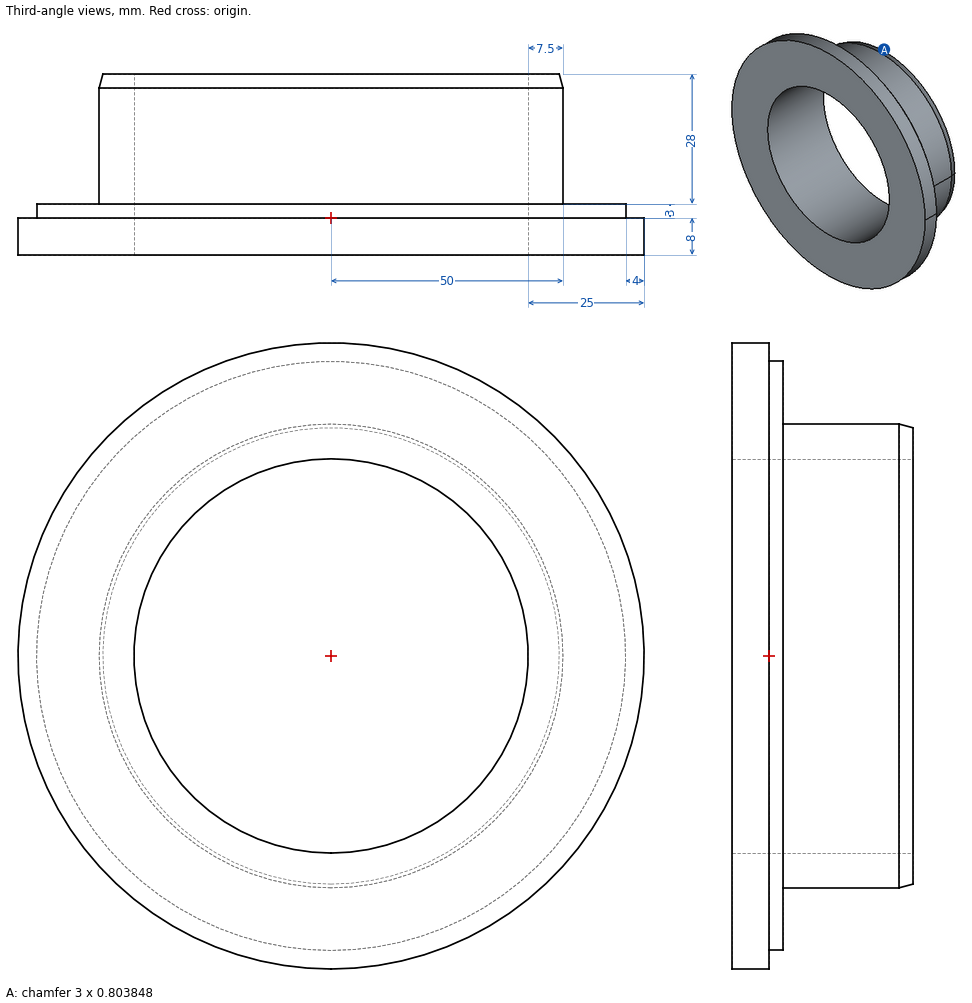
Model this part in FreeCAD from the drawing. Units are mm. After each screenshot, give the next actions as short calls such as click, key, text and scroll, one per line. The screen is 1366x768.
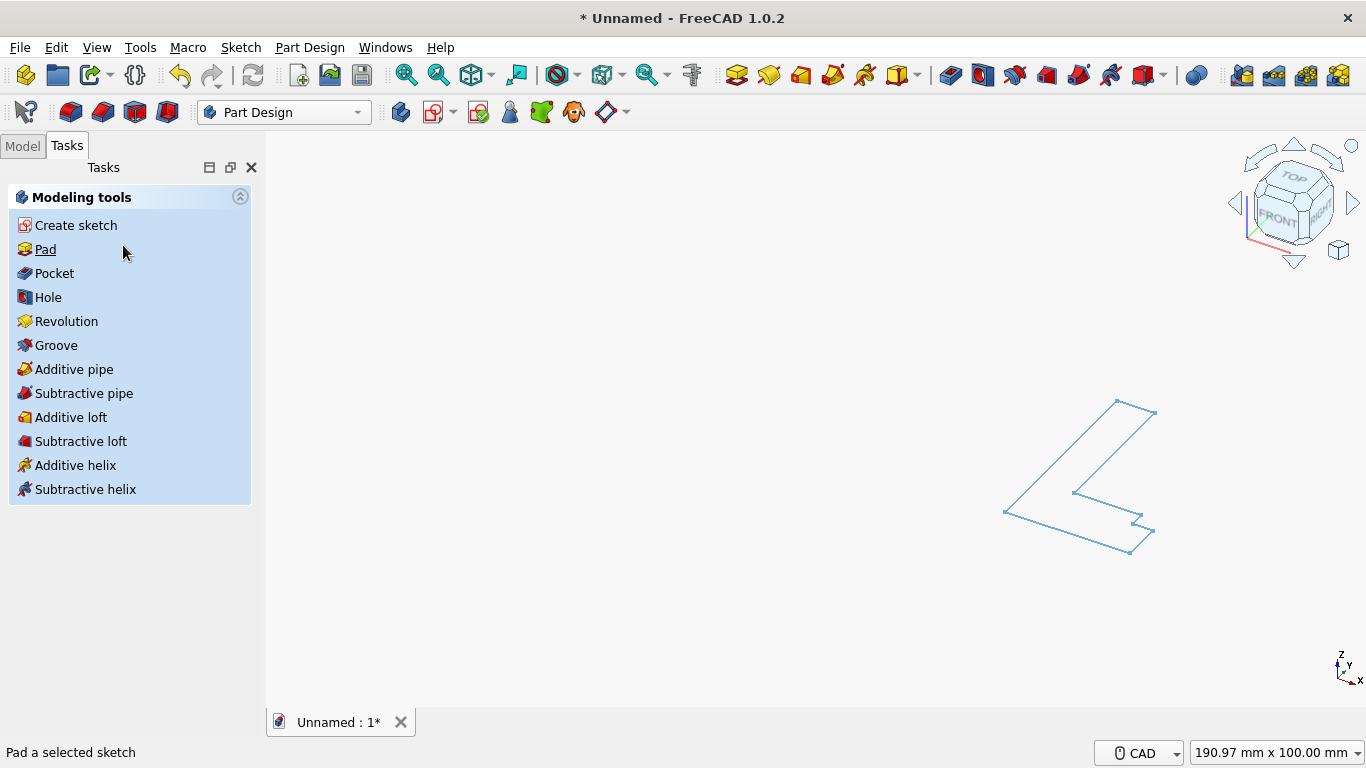
click(770, 76)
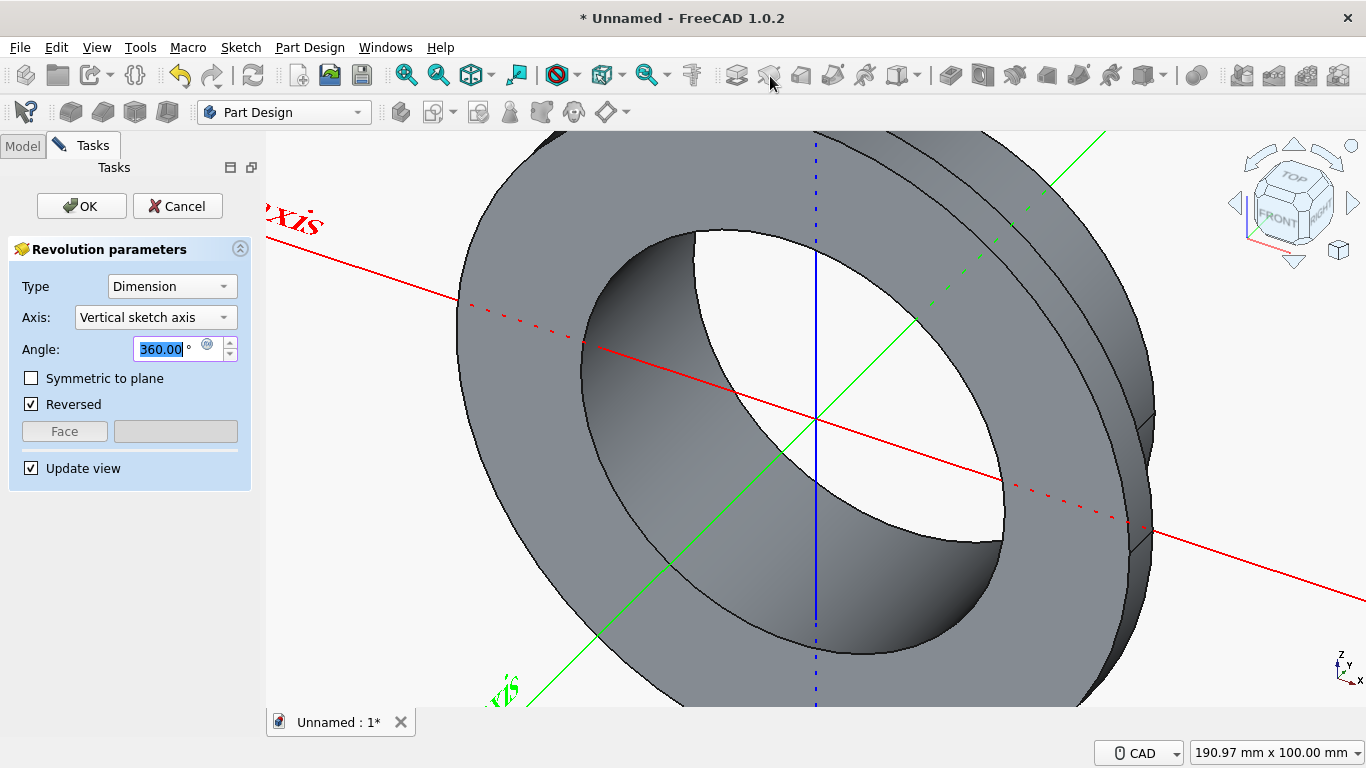
click(82, 206)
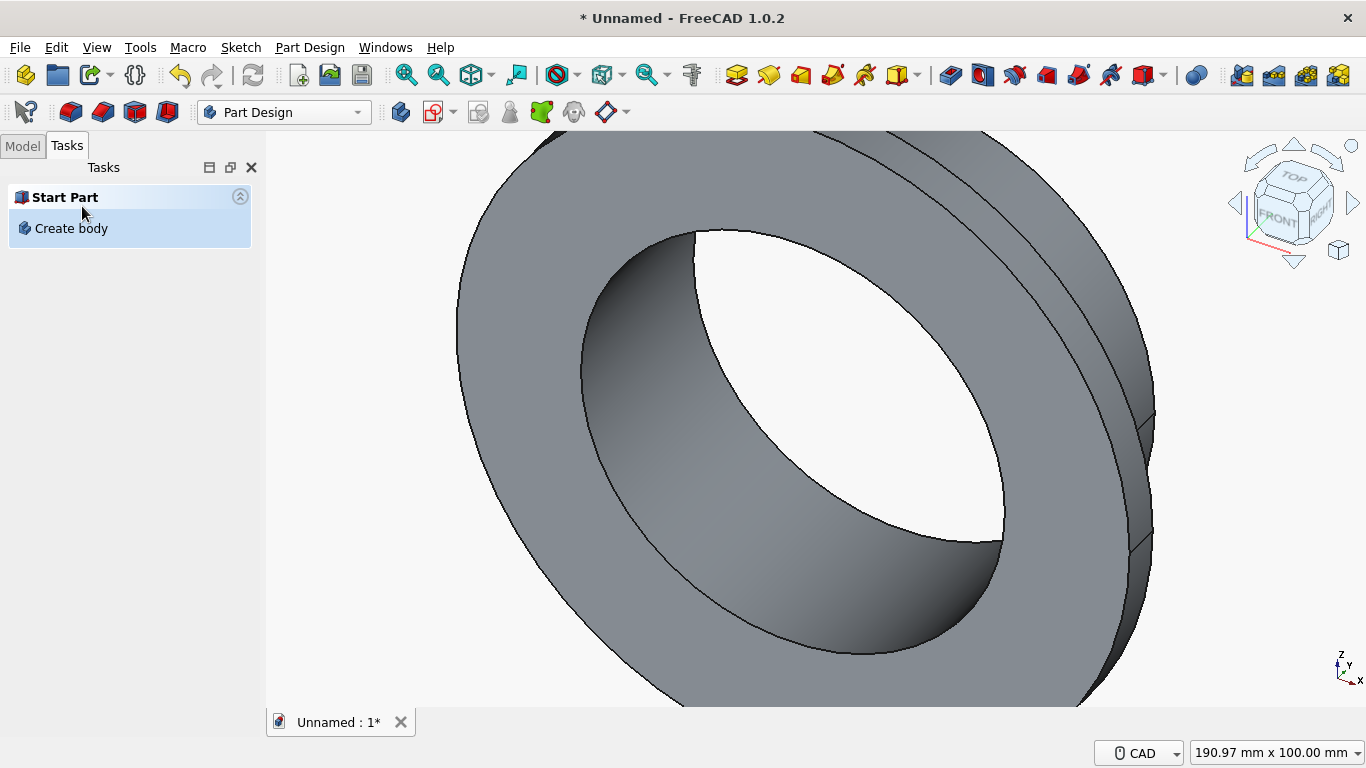
click(408, 76)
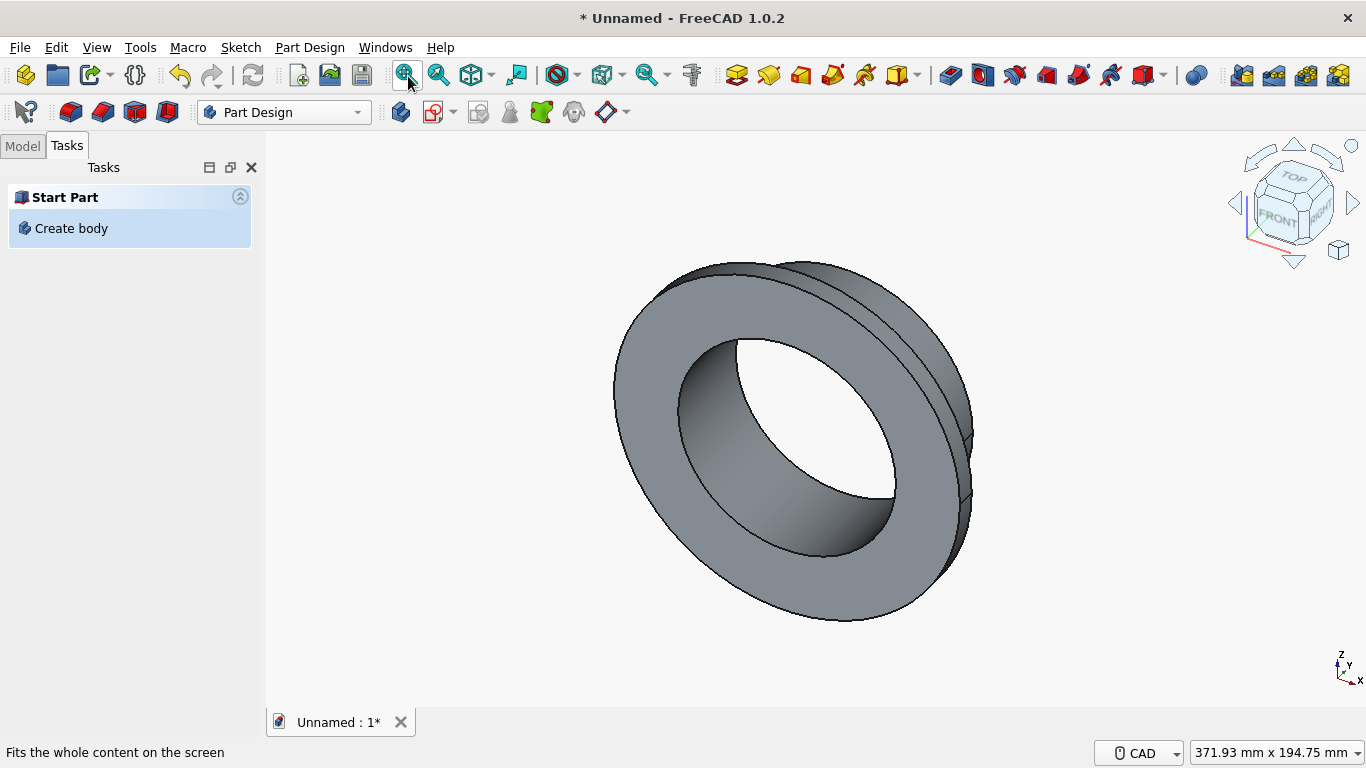
key(0)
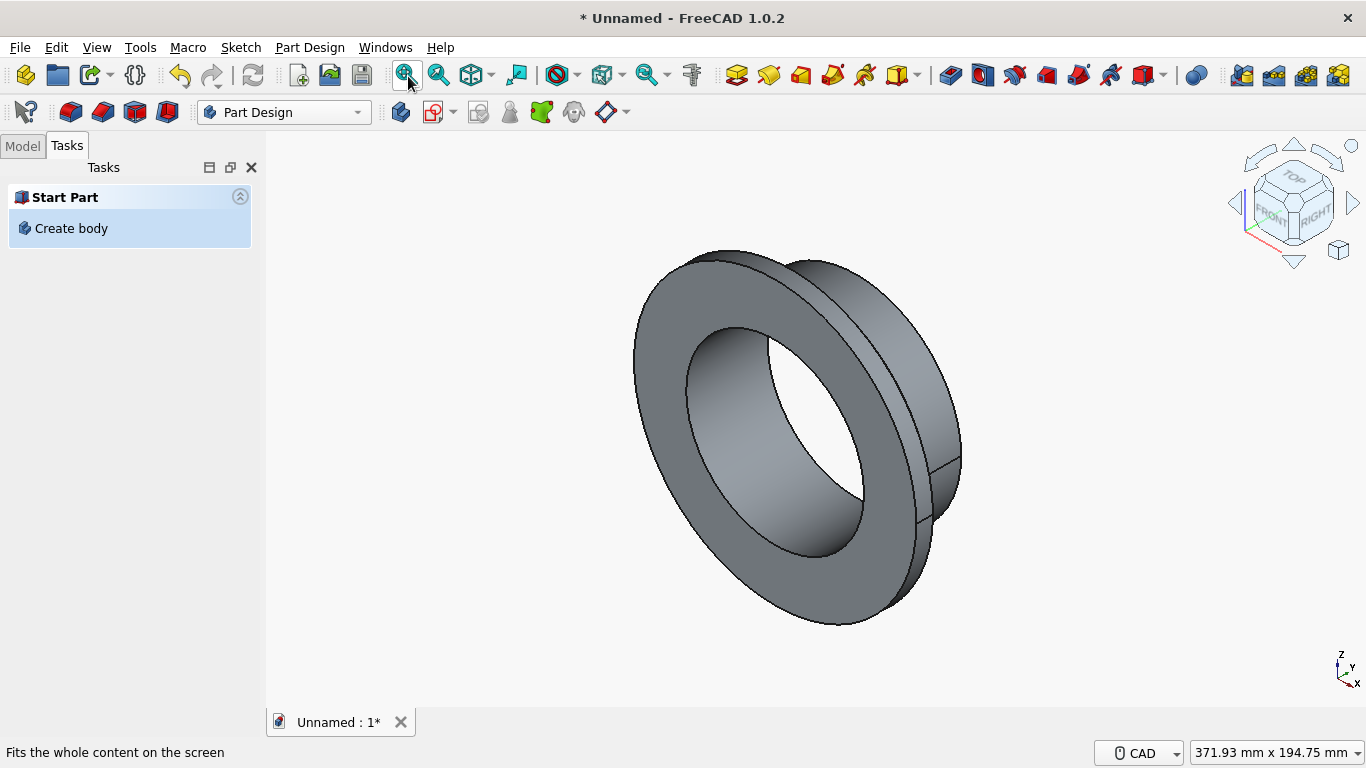
key(2)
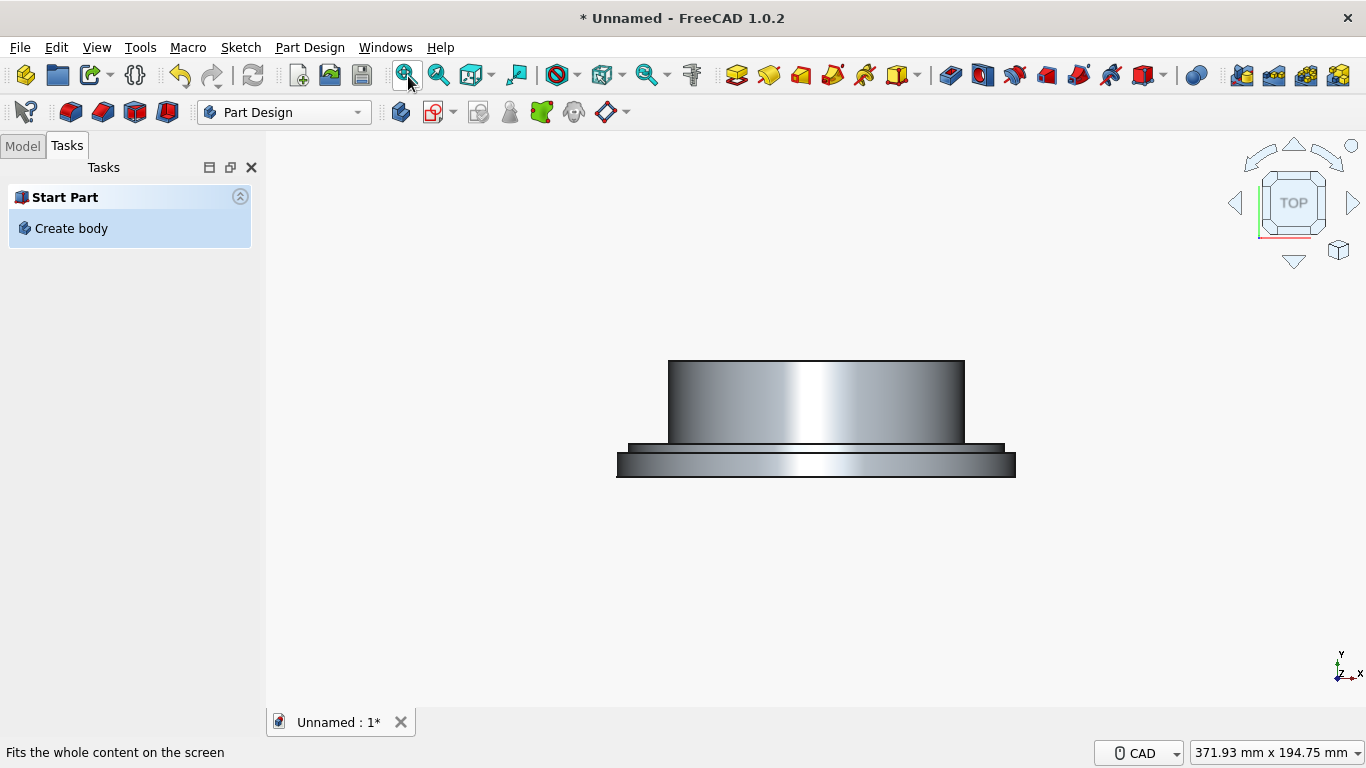
click(408, 76)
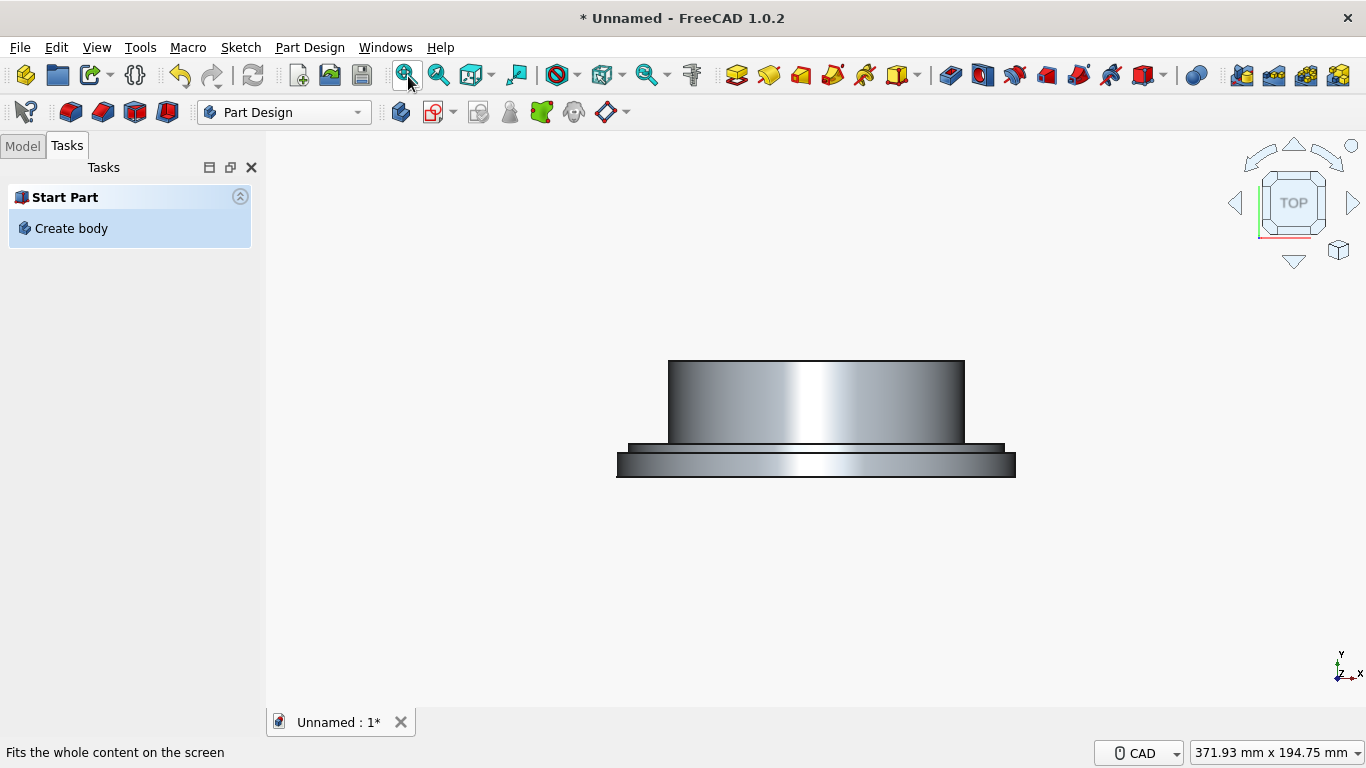
click(696, 360)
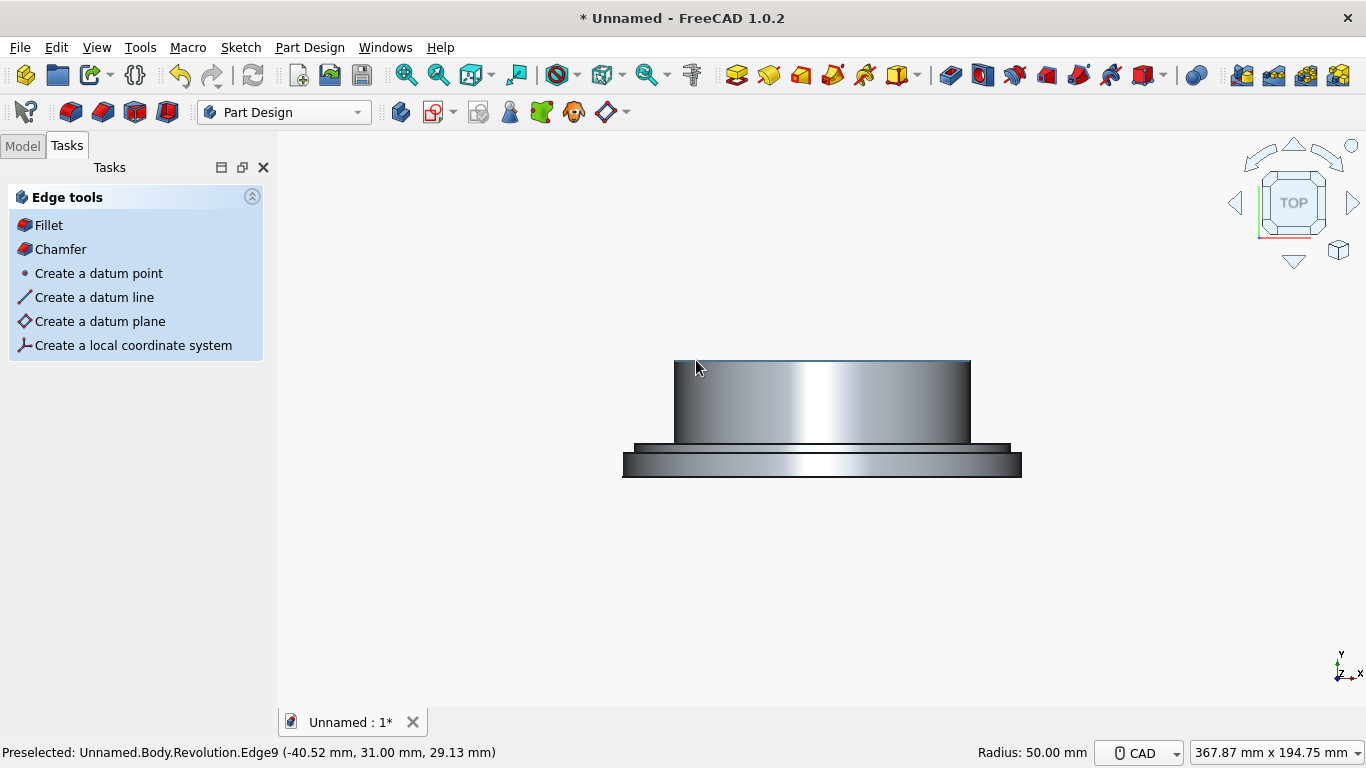
click(104, 112)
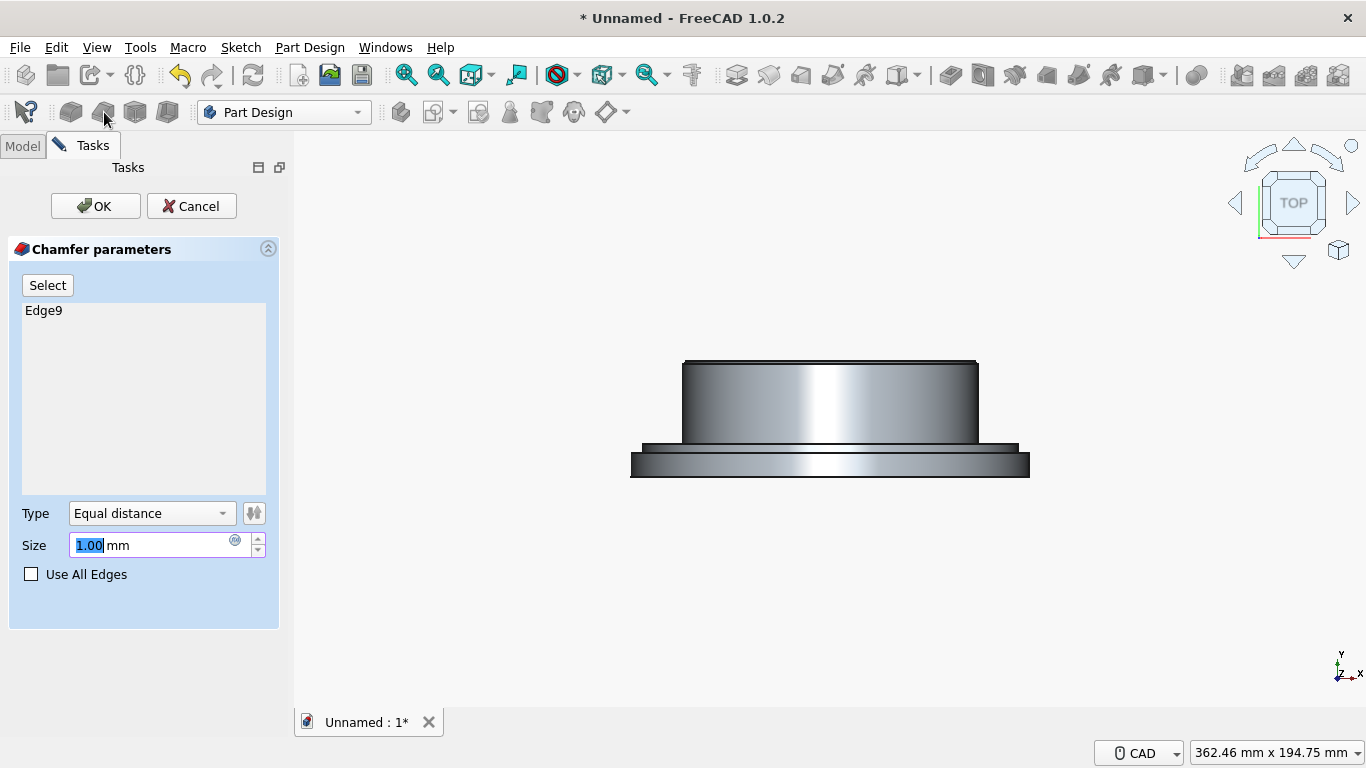
text(3)
key(Tab)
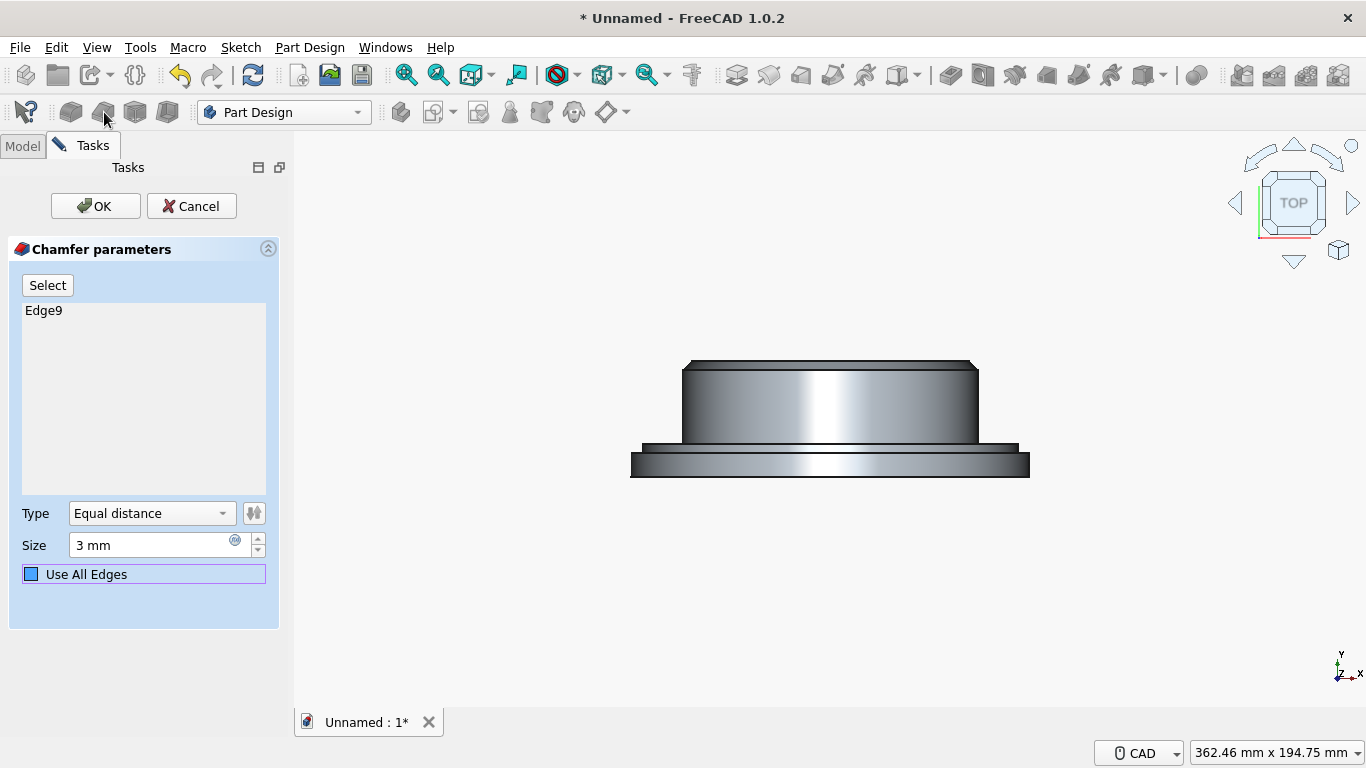
click(153, 514)